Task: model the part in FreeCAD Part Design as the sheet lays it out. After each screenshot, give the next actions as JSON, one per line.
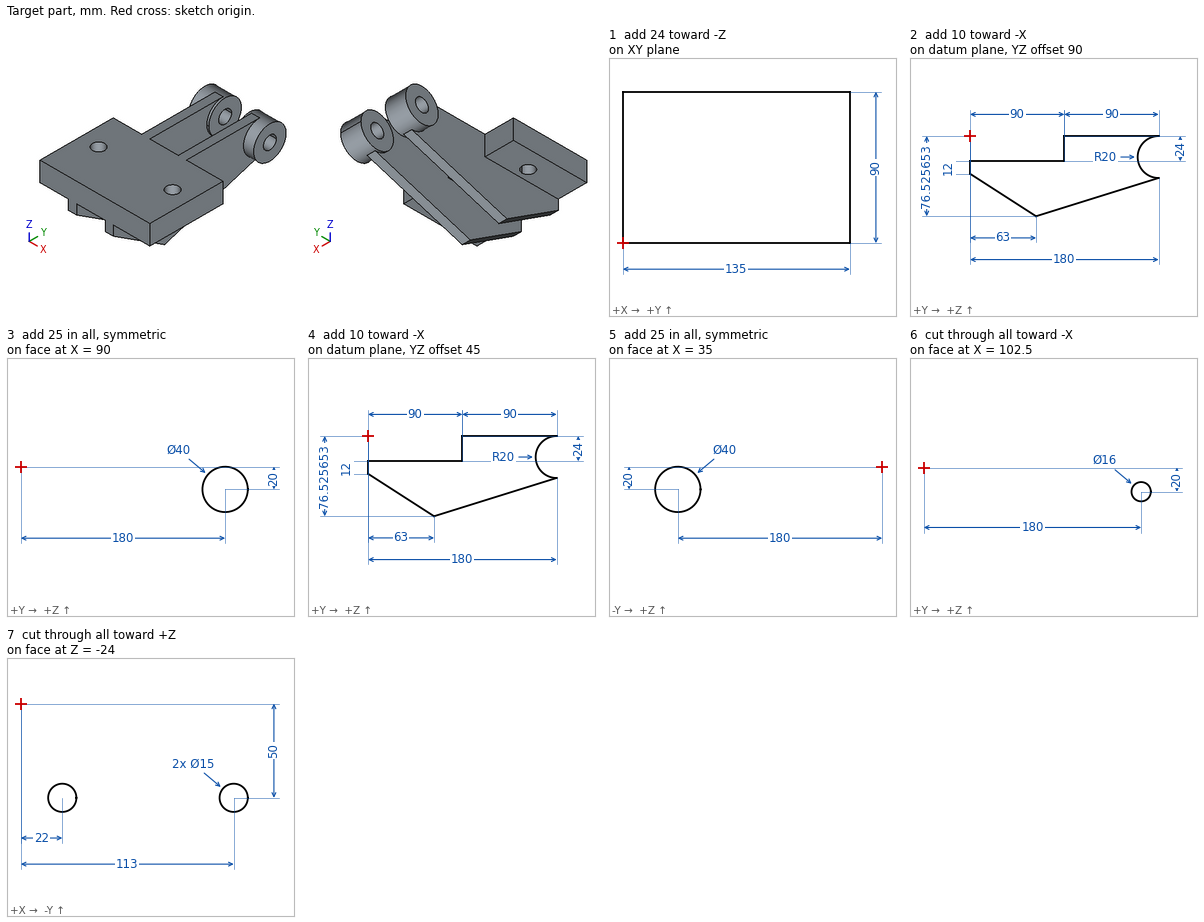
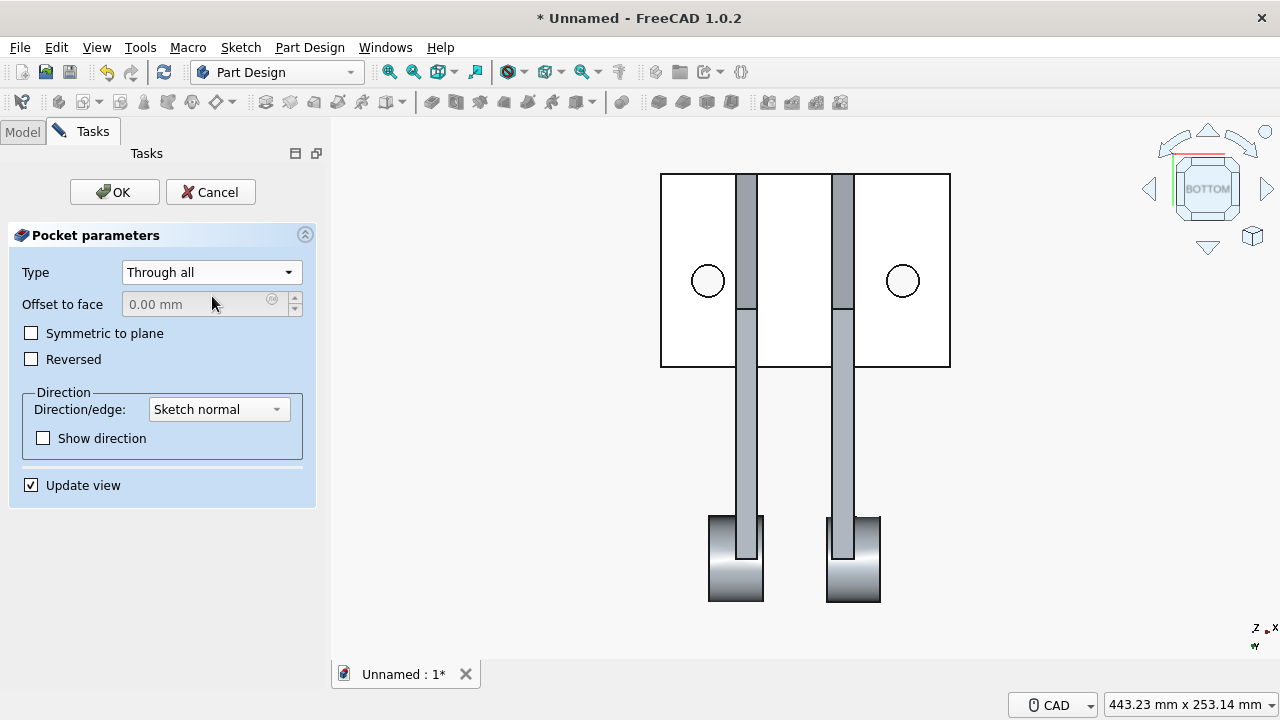
{"action": "left_click", "coordinate": [115, 192]}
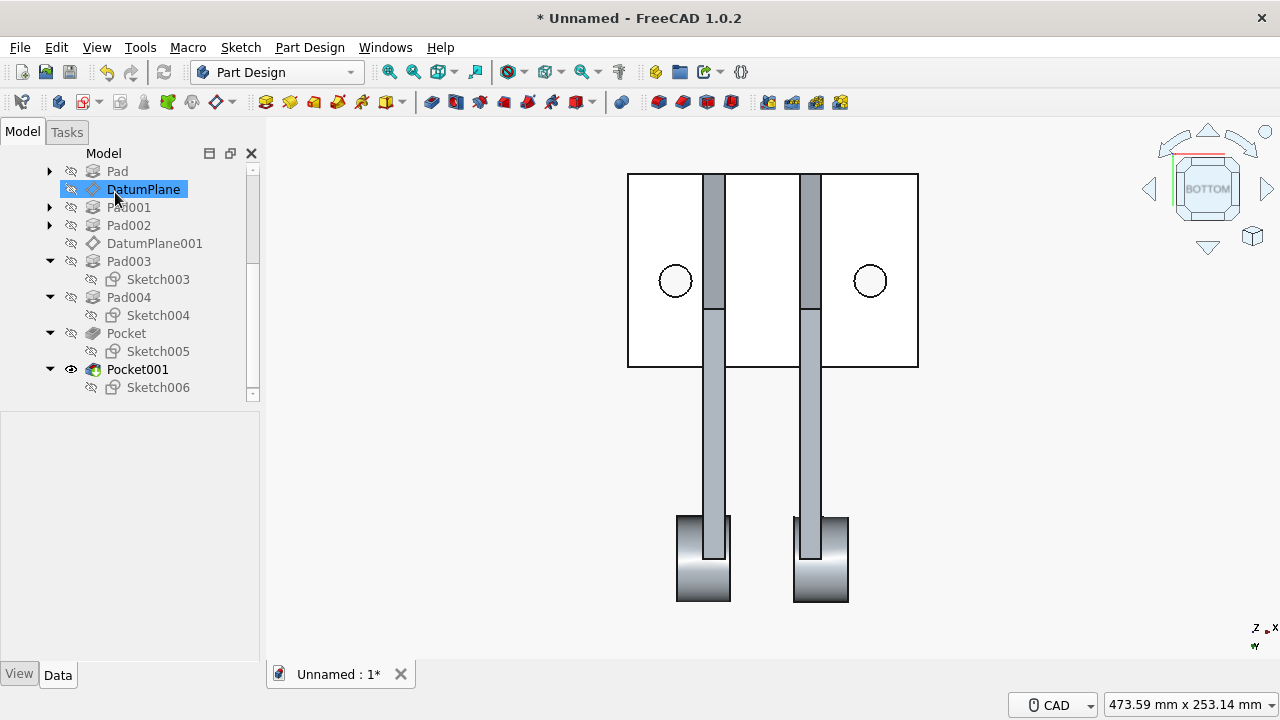
{"action": "key", "text": "0"}